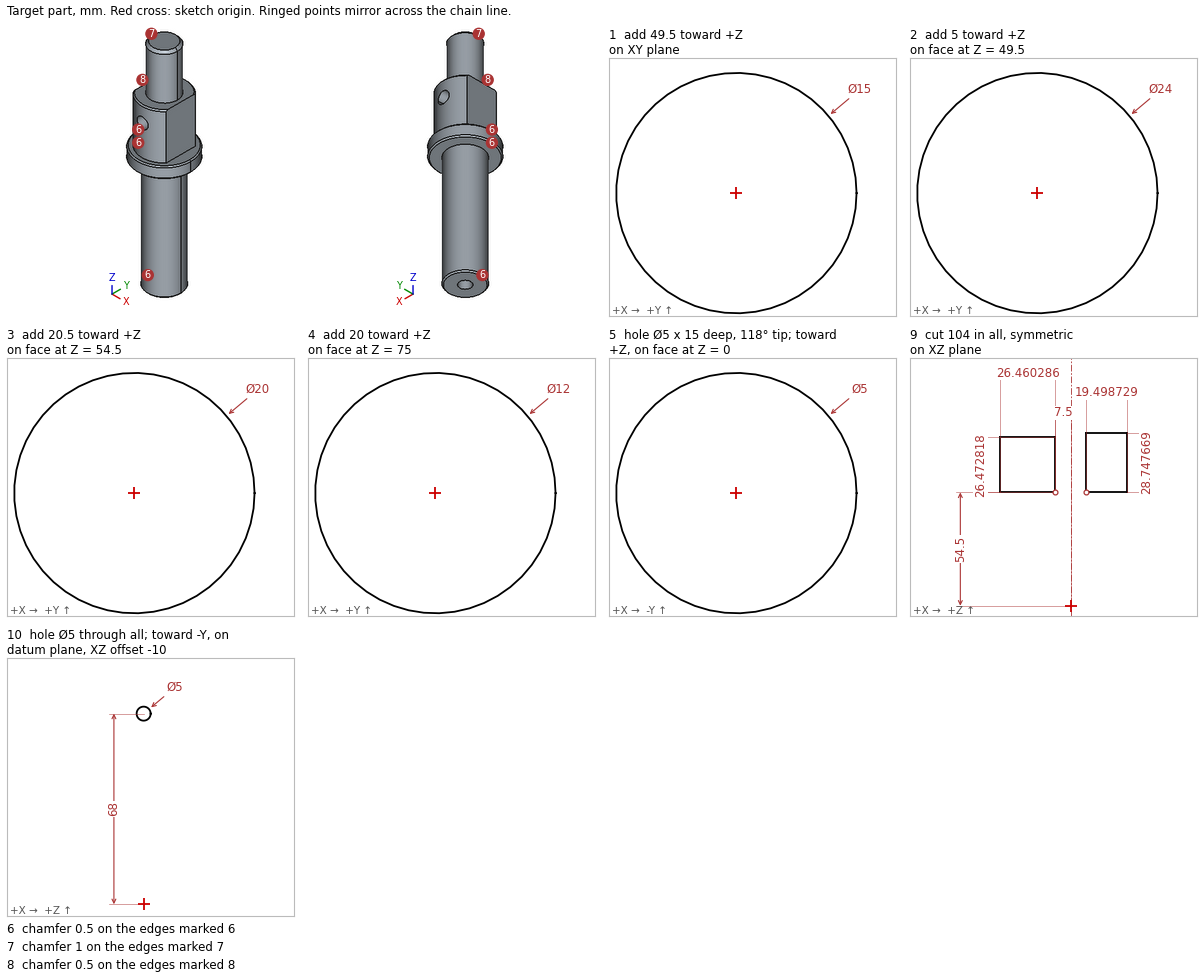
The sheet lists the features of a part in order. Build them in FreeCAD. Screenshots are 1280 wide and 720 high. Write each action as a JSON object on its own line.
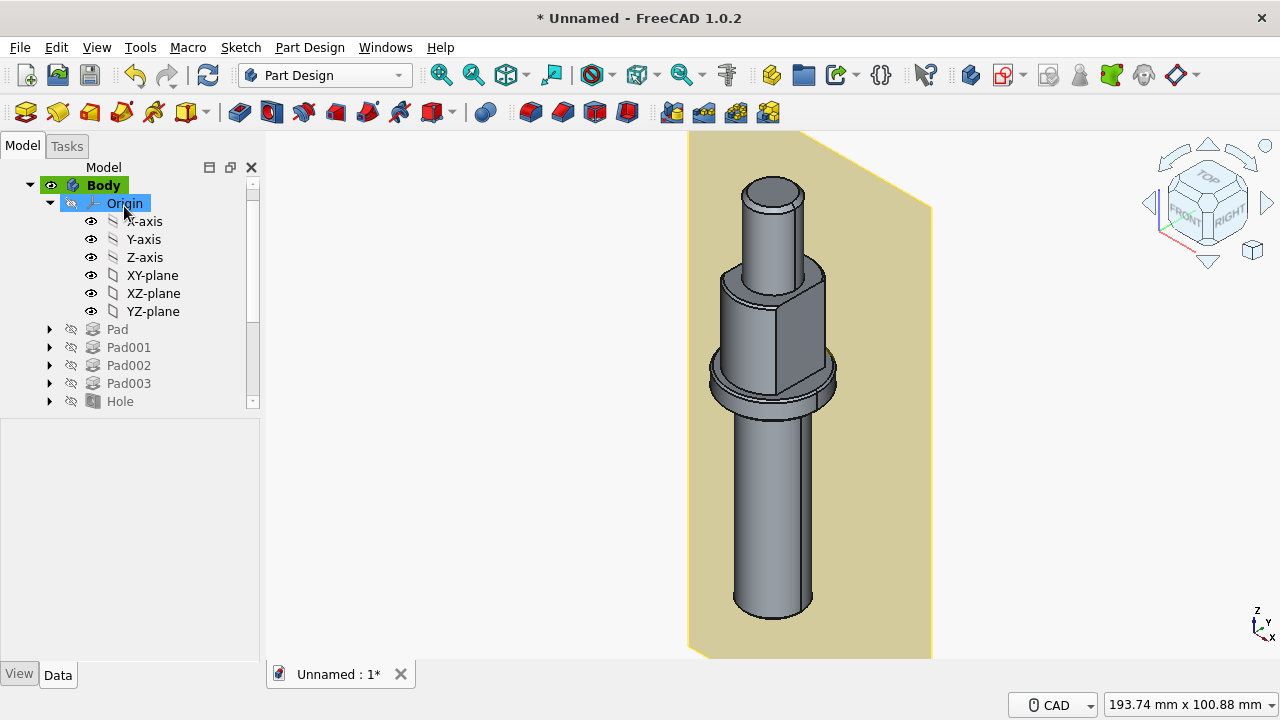
{"action": "scroll", "coordinate": [120, 289], "scroll_direction": "down", "scroll_amount": 3}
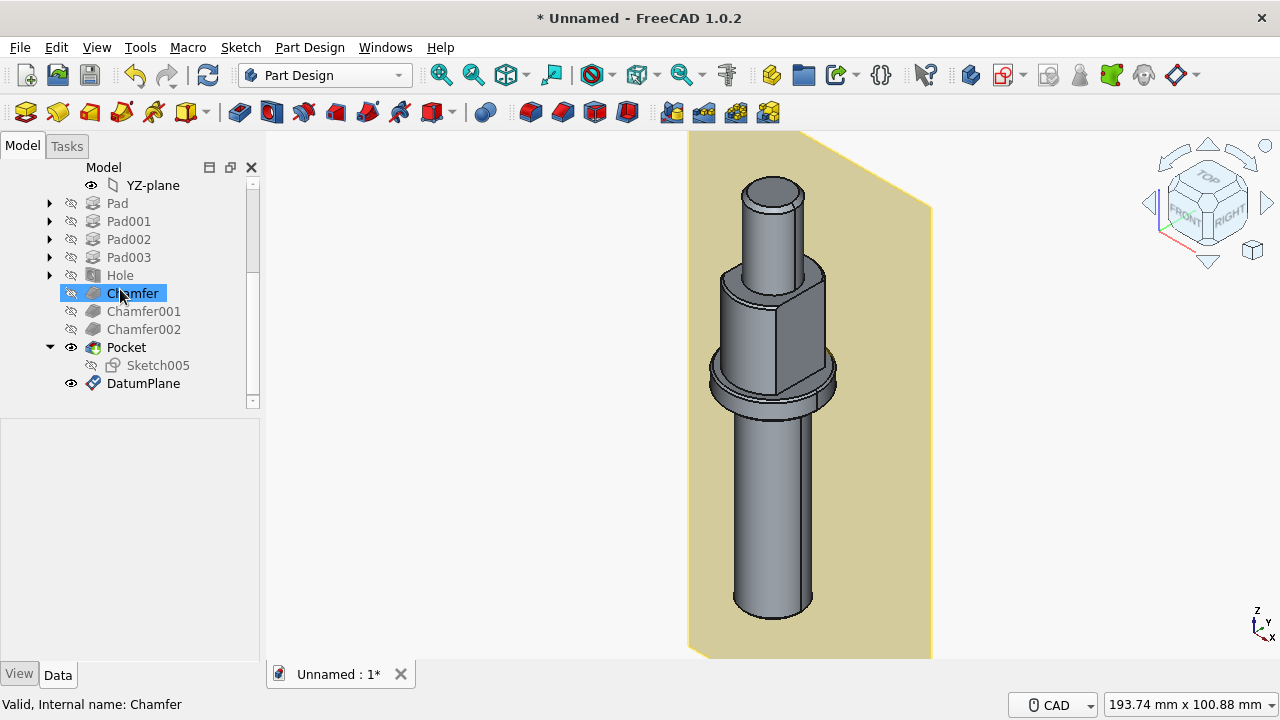
{"action": "left_click", "coordinate": [116, 383]}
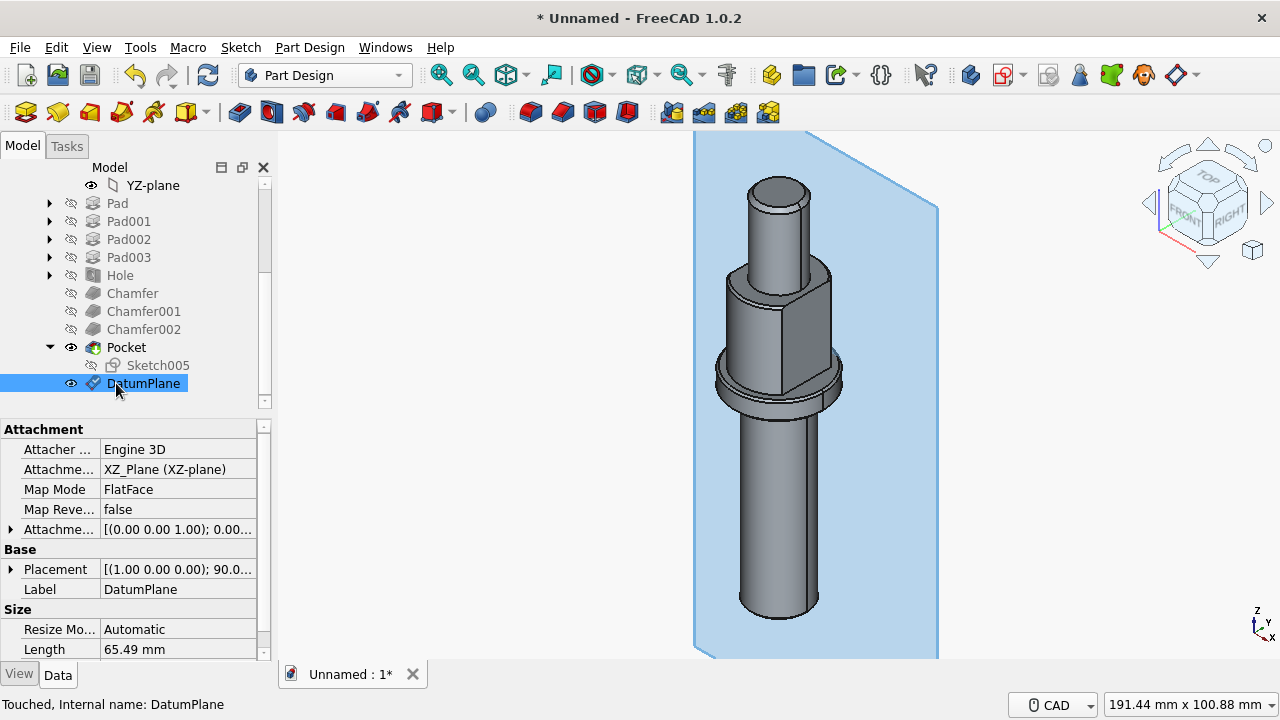
{"action": "left_click", "coordinate": [1004, 76]}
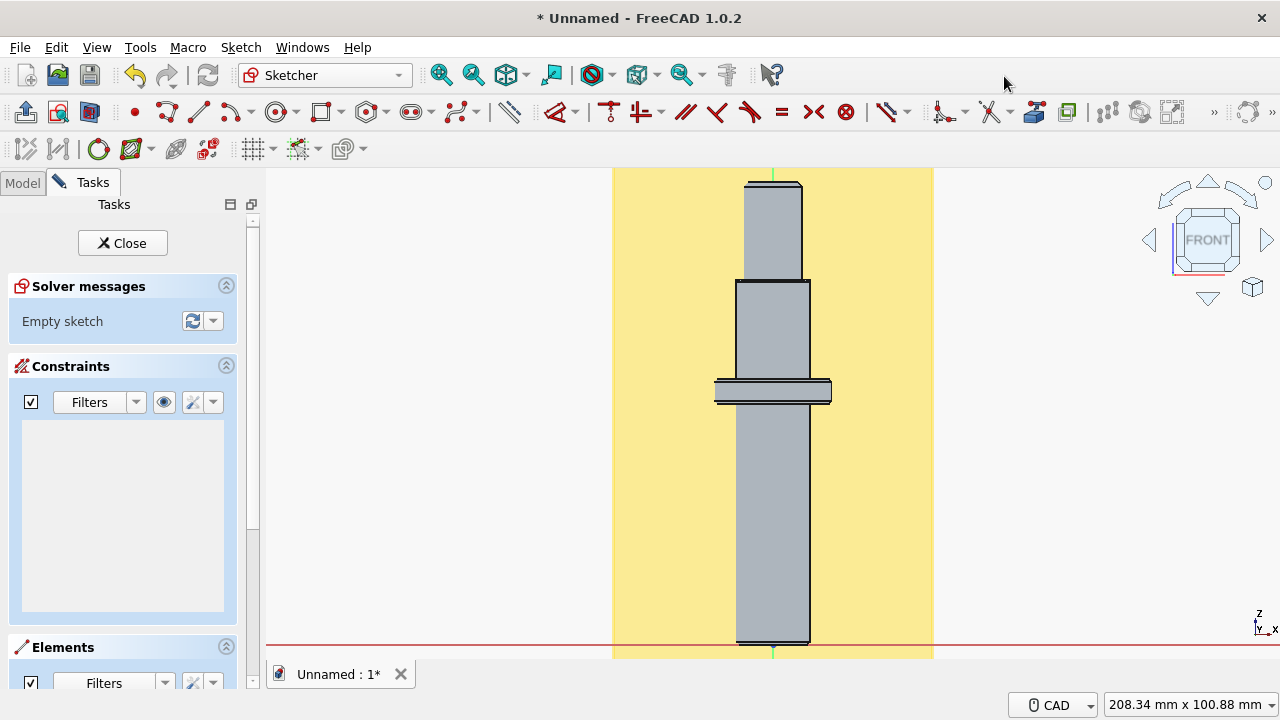
{"action": "key", "text": "q s"}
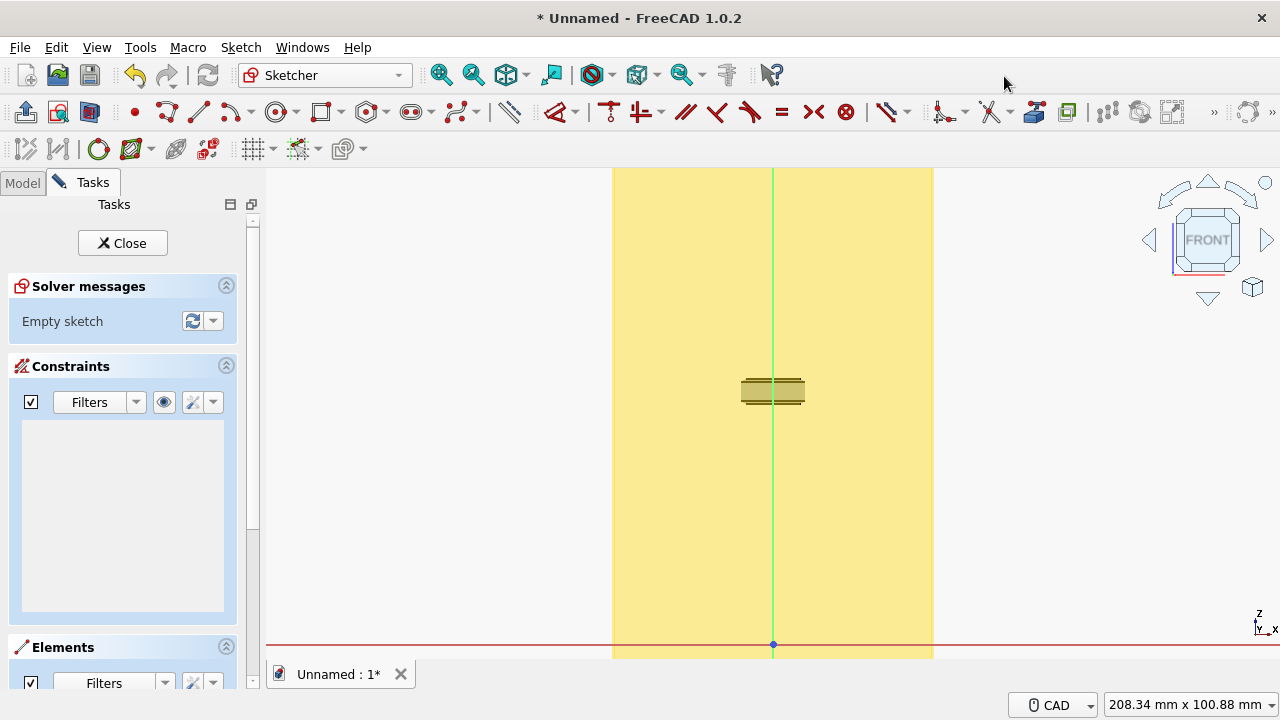
{"action": "scroll", "coordinate": [778, 306], "scroll_direction": "up", "scroll_amount": 13}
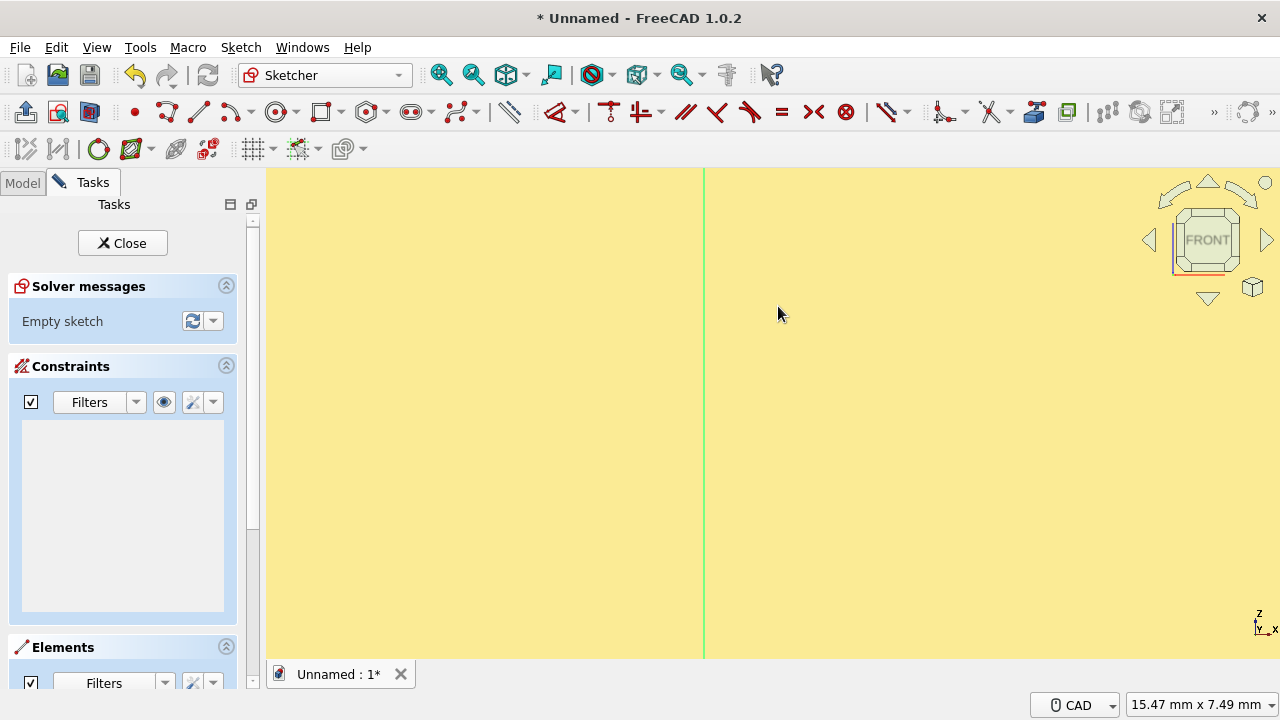
{"action": "key", "text": "g c"}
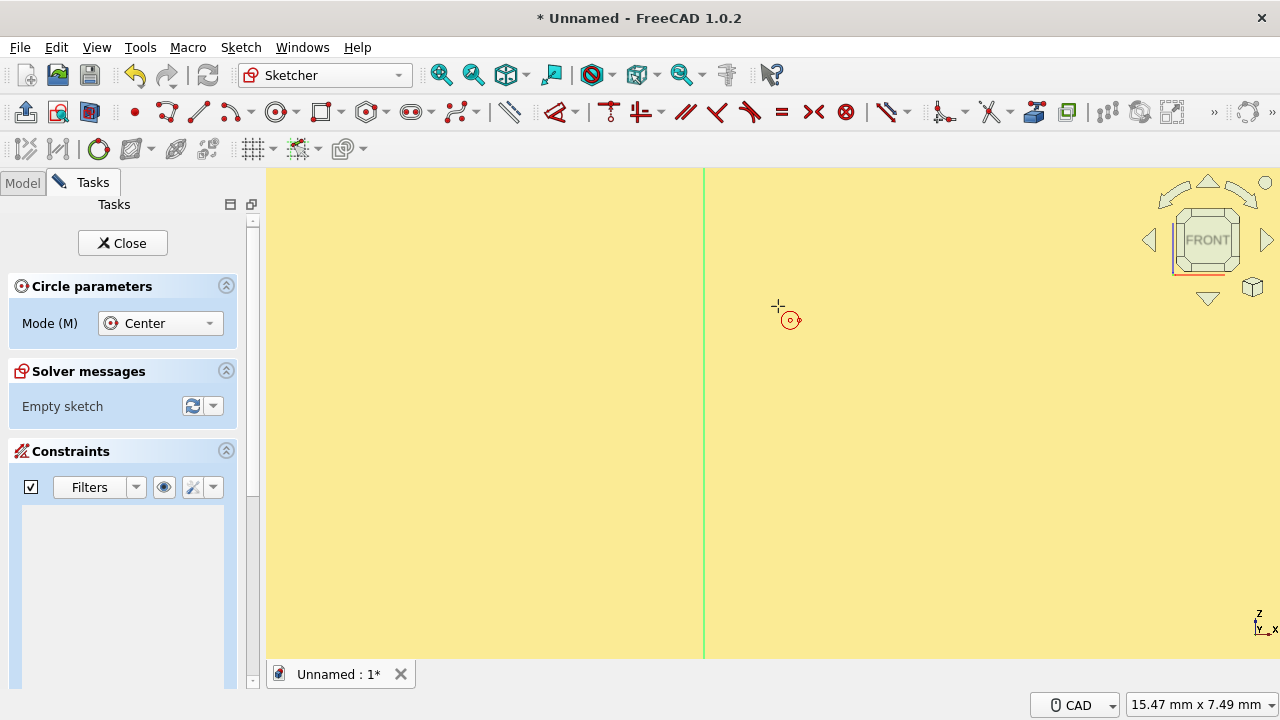
{"action": "left_click", "coordinate": [704, 406]}
{"action": "mouse_move", "coordinate": [820, 291]}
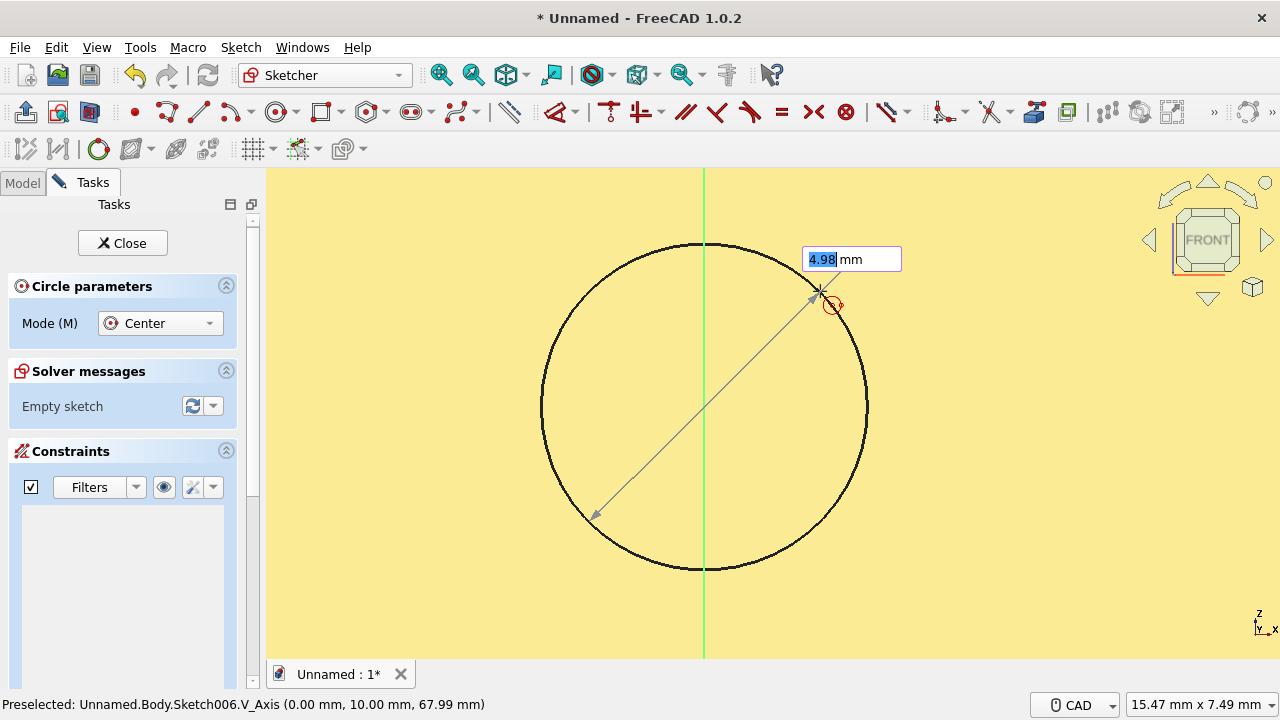
{"action": "type", "text": "5"}
{"action": "key", "text": "Return"}
{"action": "key", "text": "Escape"}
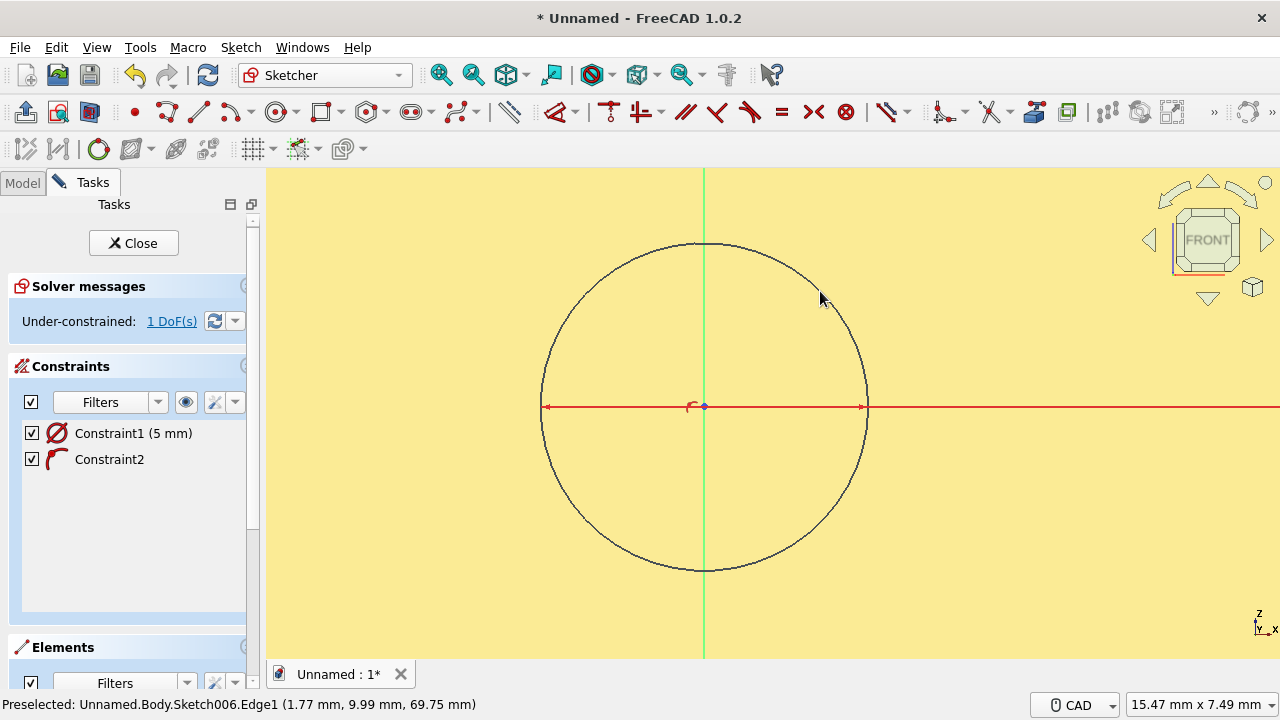
{"action": "key", "text": "d"}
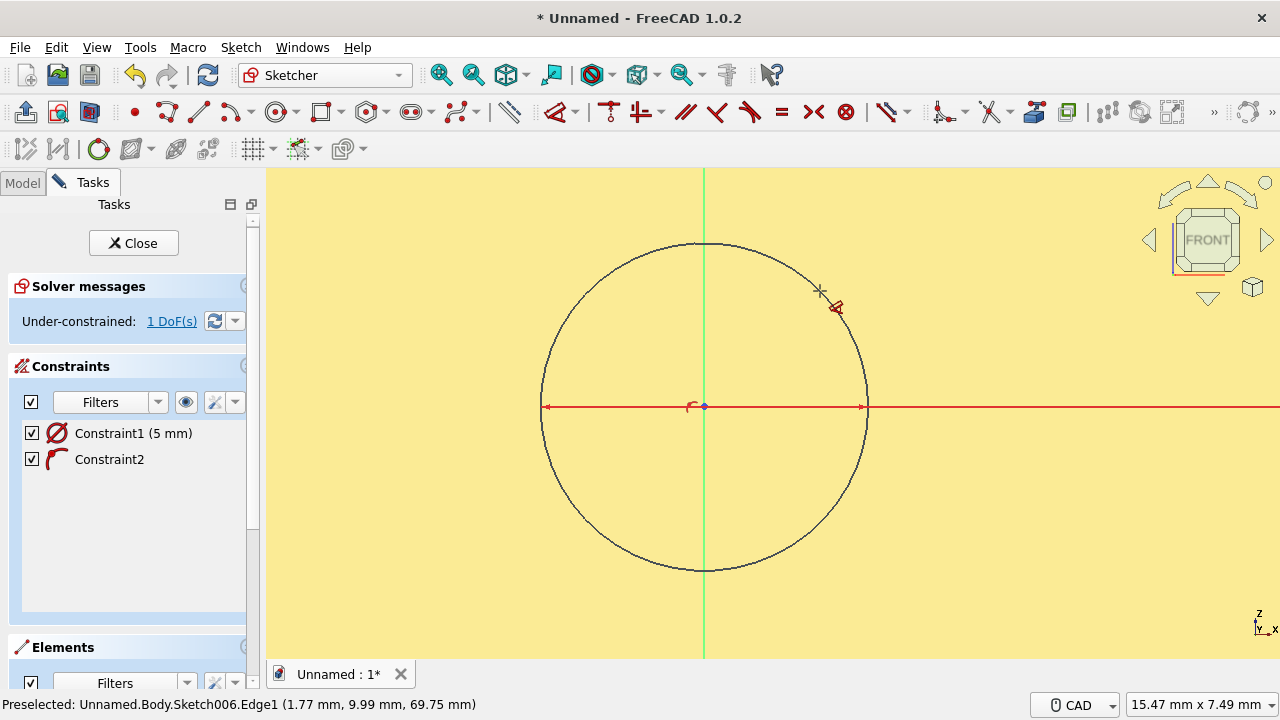
{"action": "left_click", "coordinate": [704, 407]}
{"action": "left_click", "coordinate": [738, 519]}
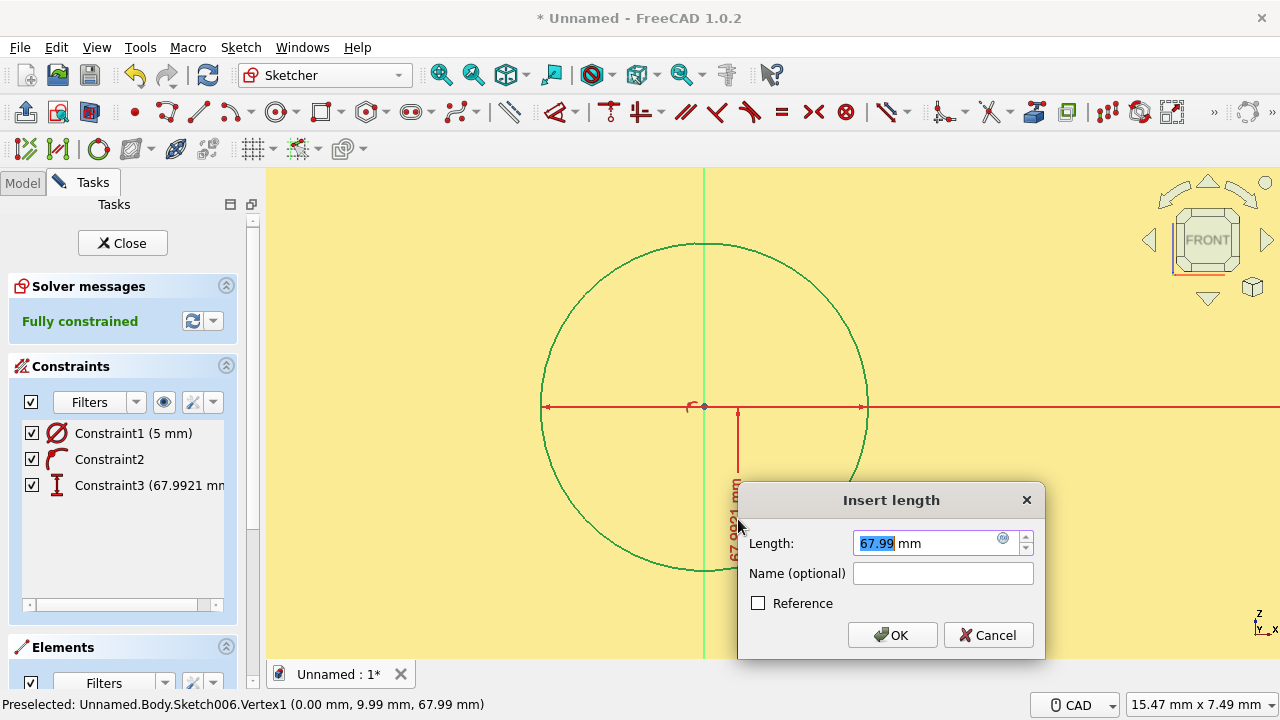
{"action": "type", "text": "68"}
{"action": "key", "text": "Return"}
{"action": "key", "text": "Escape"}